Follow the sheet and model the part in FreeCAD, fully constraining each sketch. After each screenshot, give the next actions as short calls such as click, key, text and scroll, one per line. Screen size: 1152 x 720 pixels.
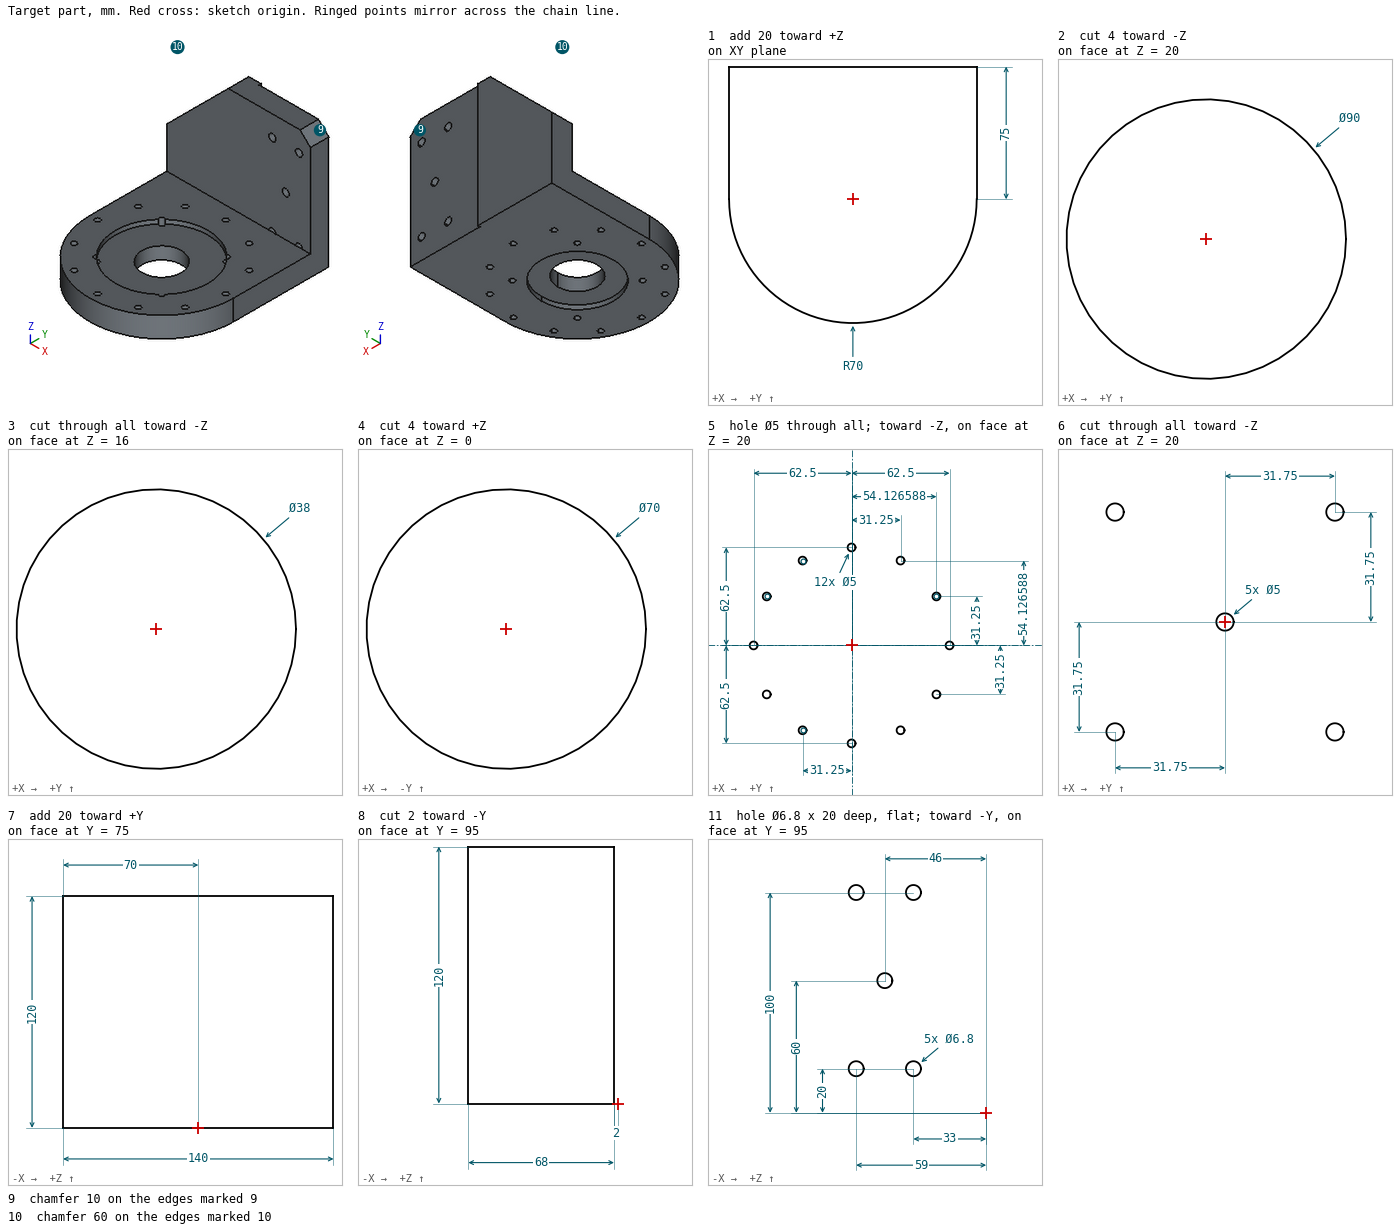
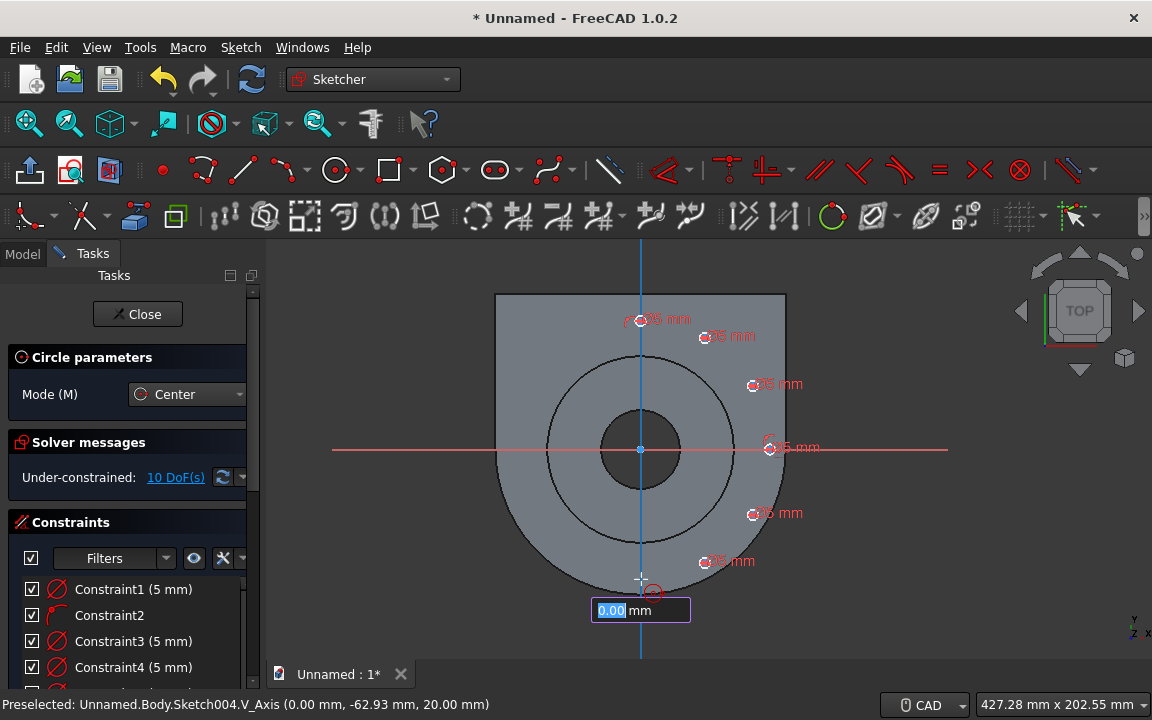
scroll(645, 577, up, 6)
move(645, 576)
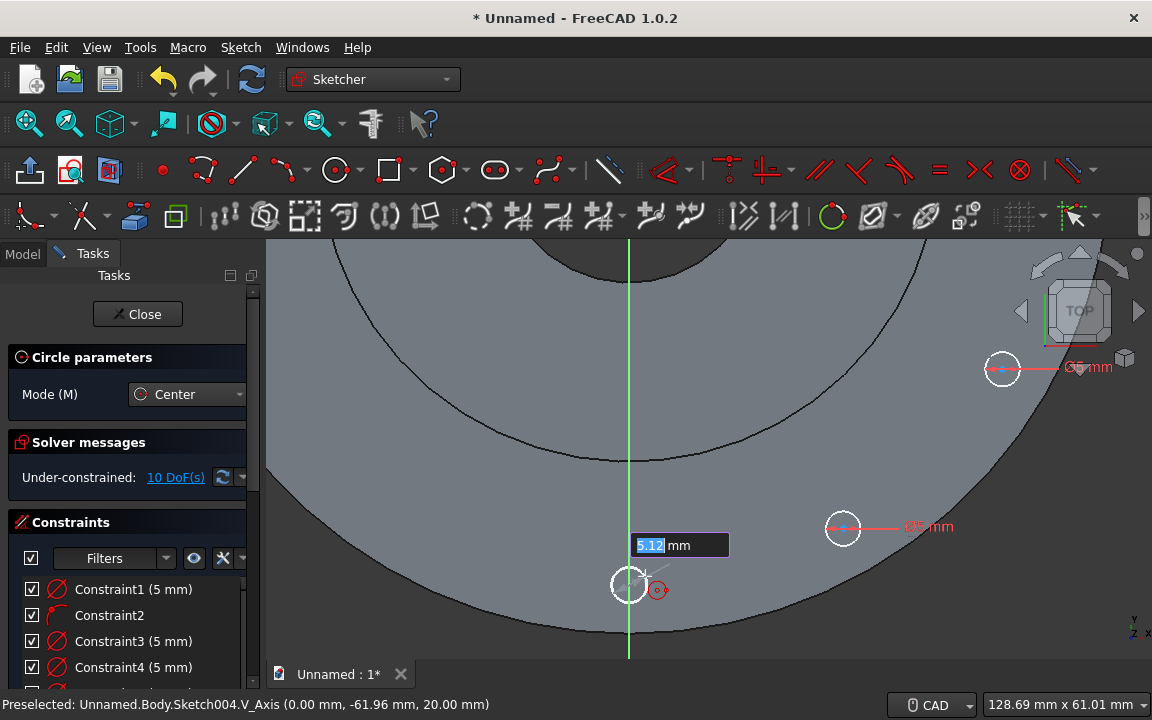
text(5)
key(Return)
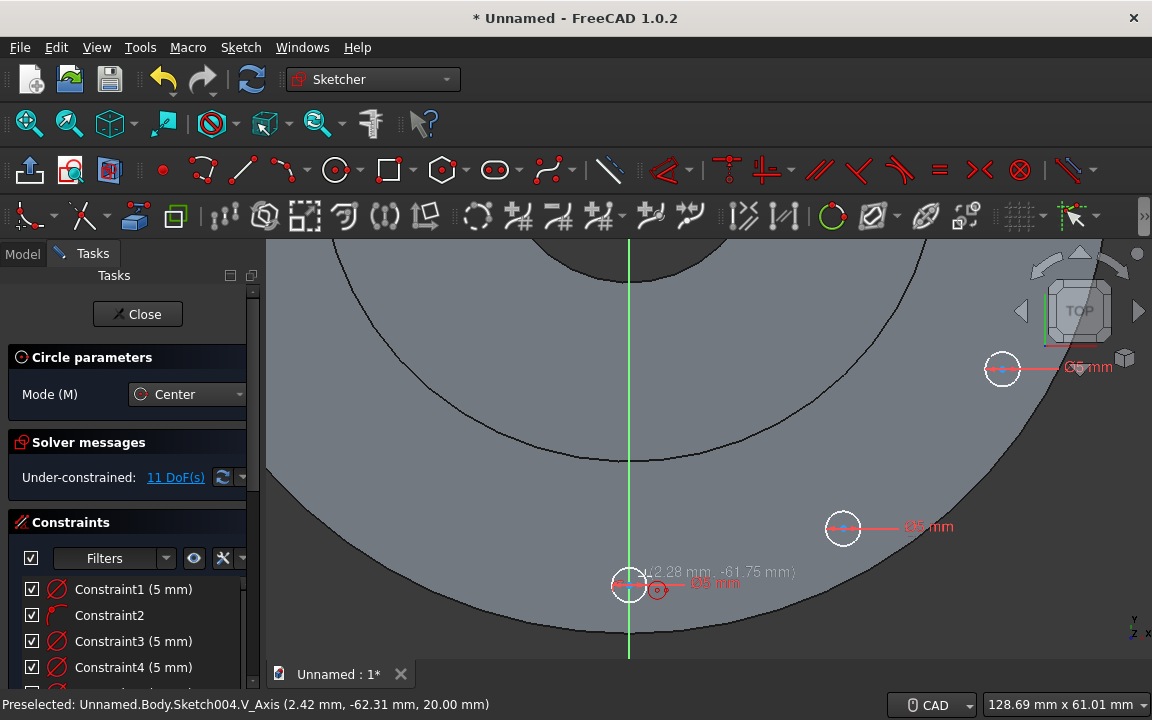
scroll(414, 524, up, 2)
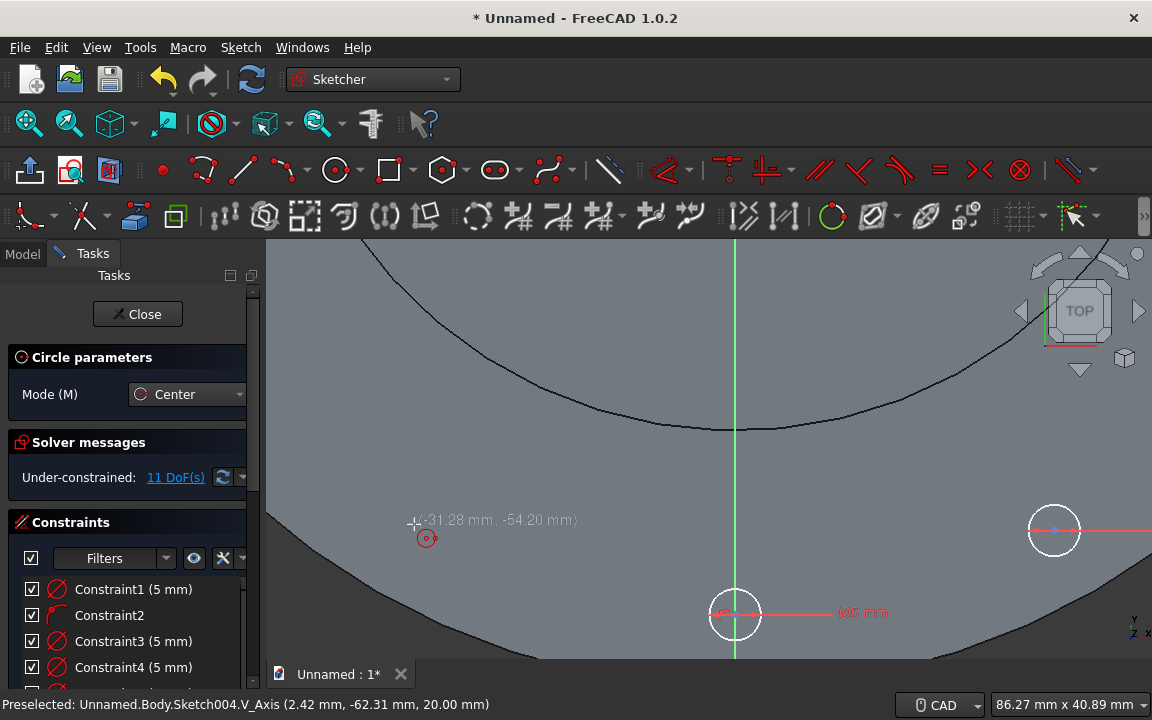
scroll(617, 571, down, 8)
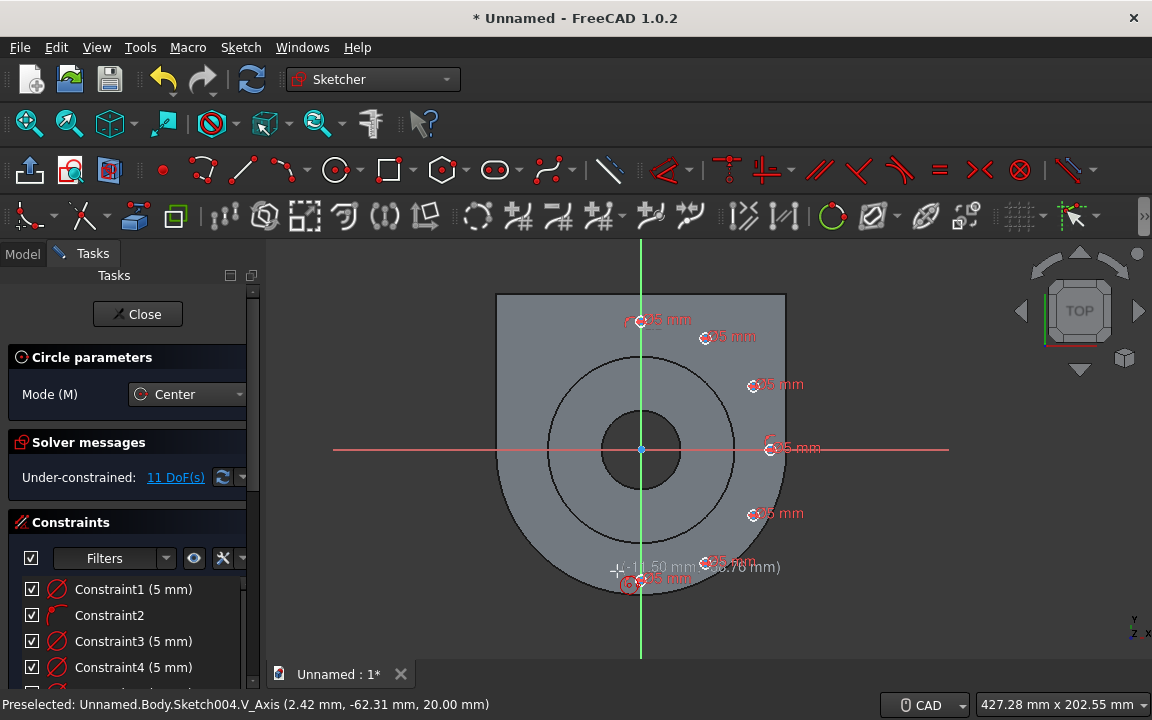
click(576, 562)
move(580, 559)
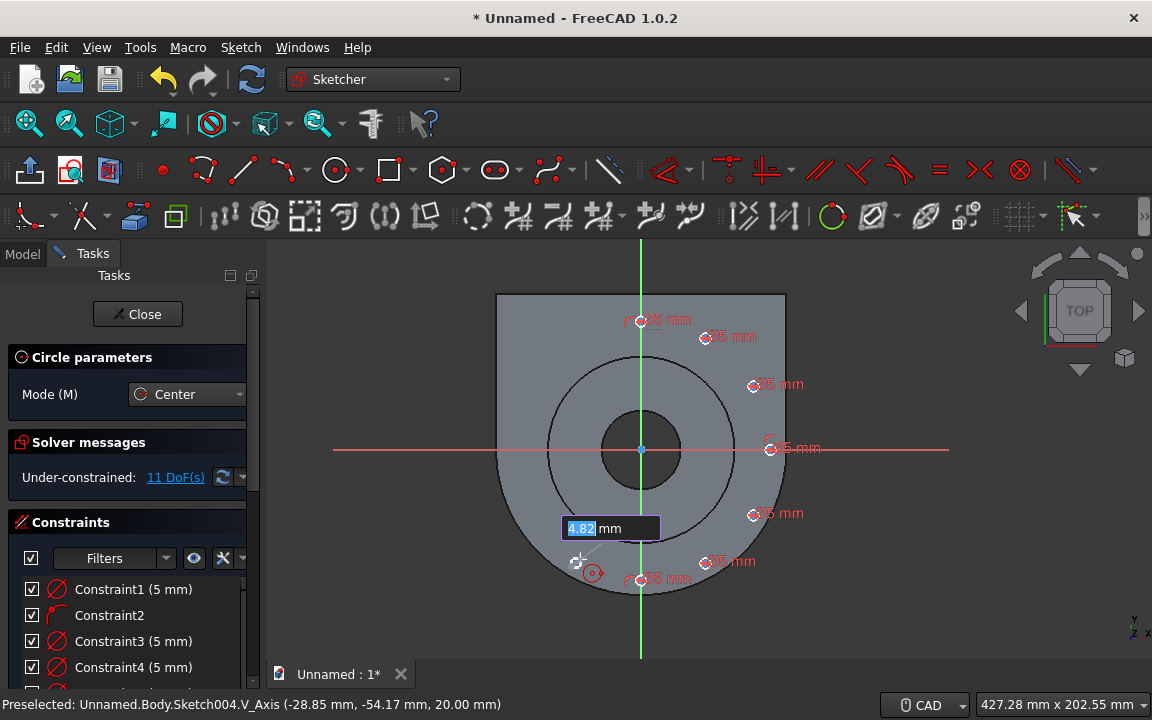
text(5)
key(Return)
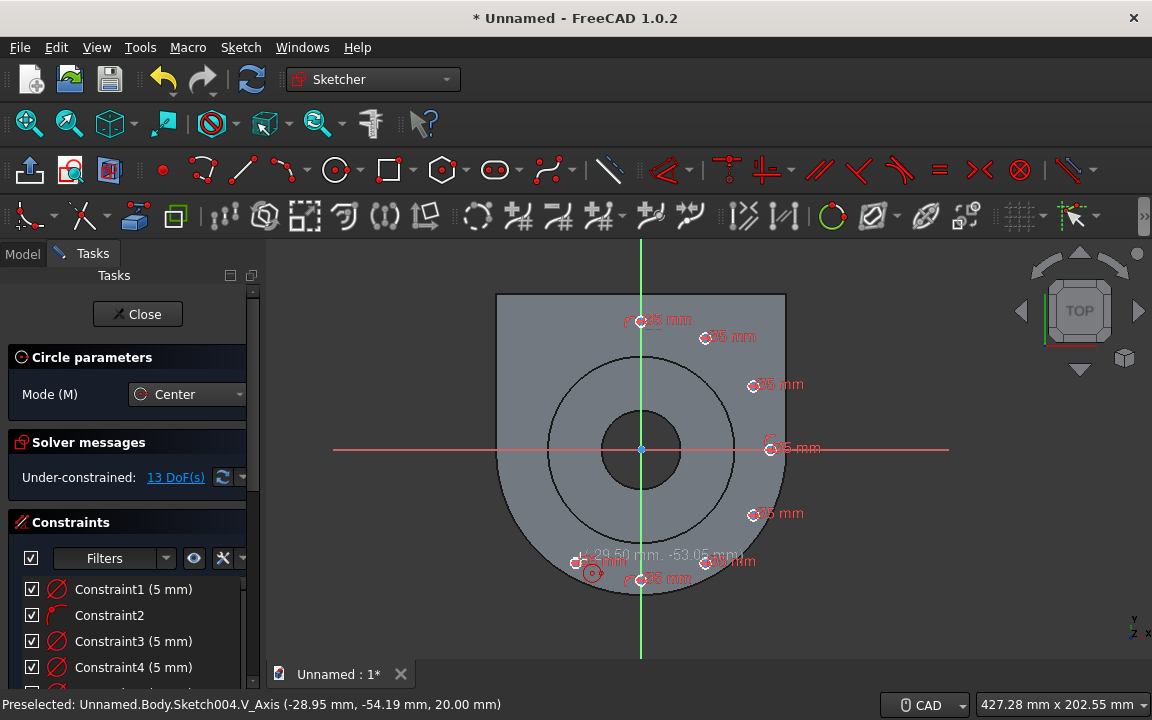
scroll(529, 515, up, 8)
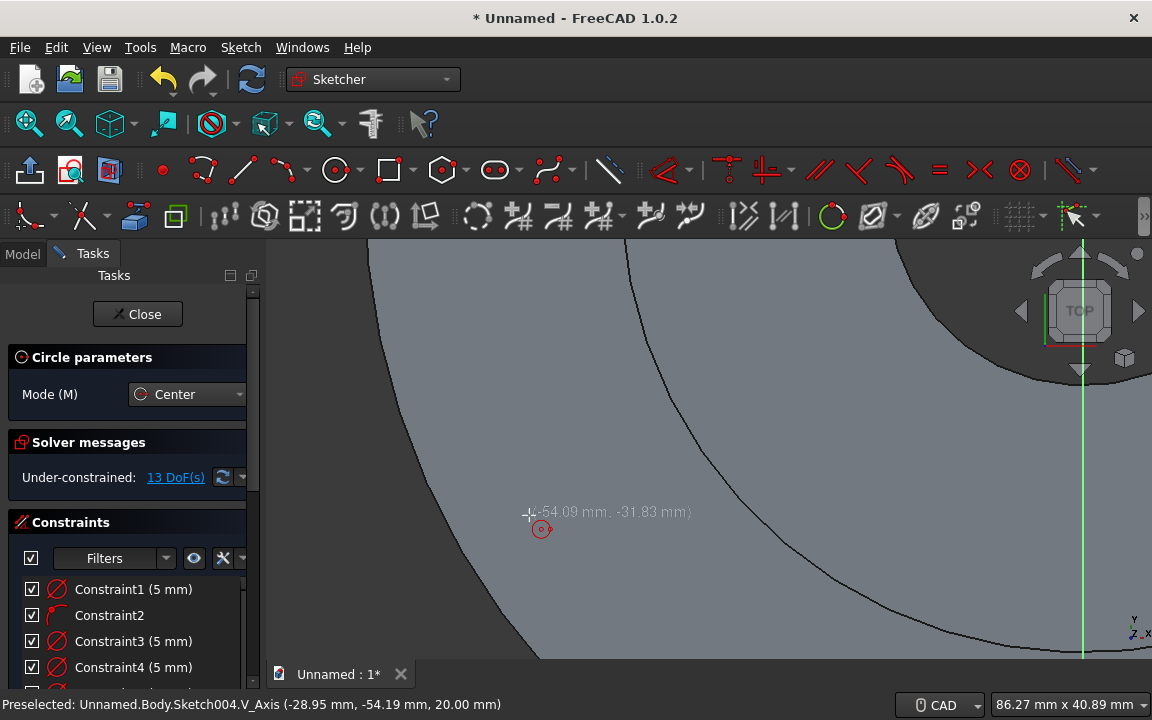
scroll(528, 514, down, 8)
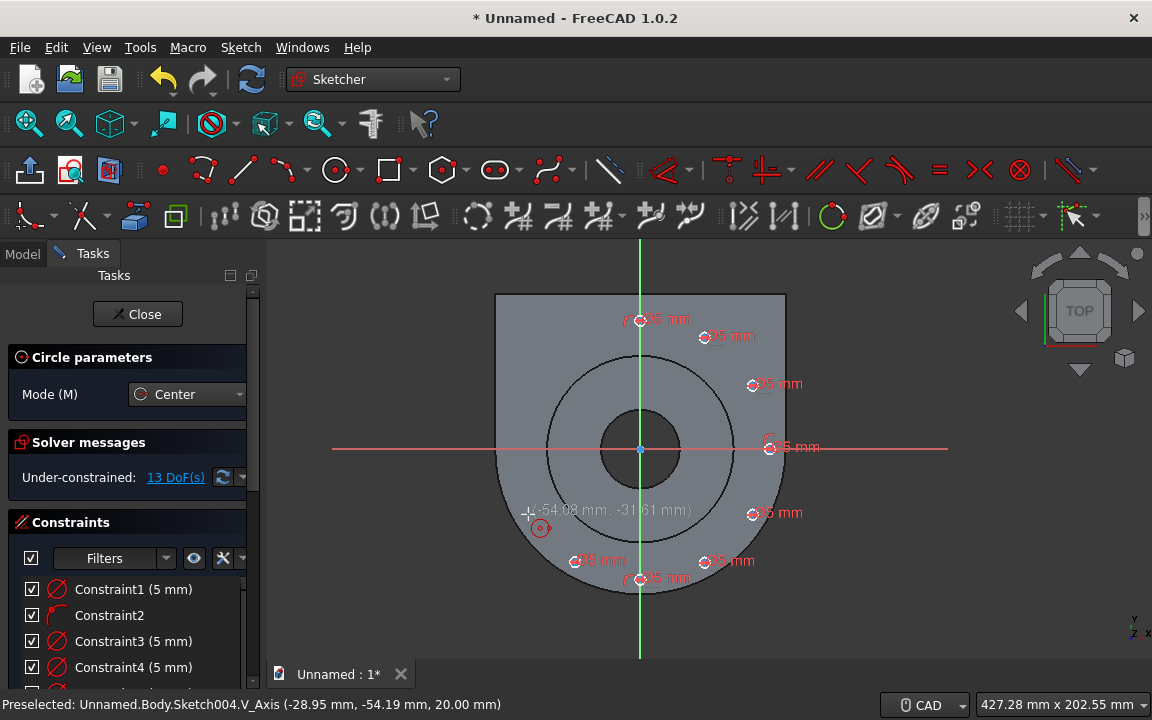
click(528, 514)
move(532, 510)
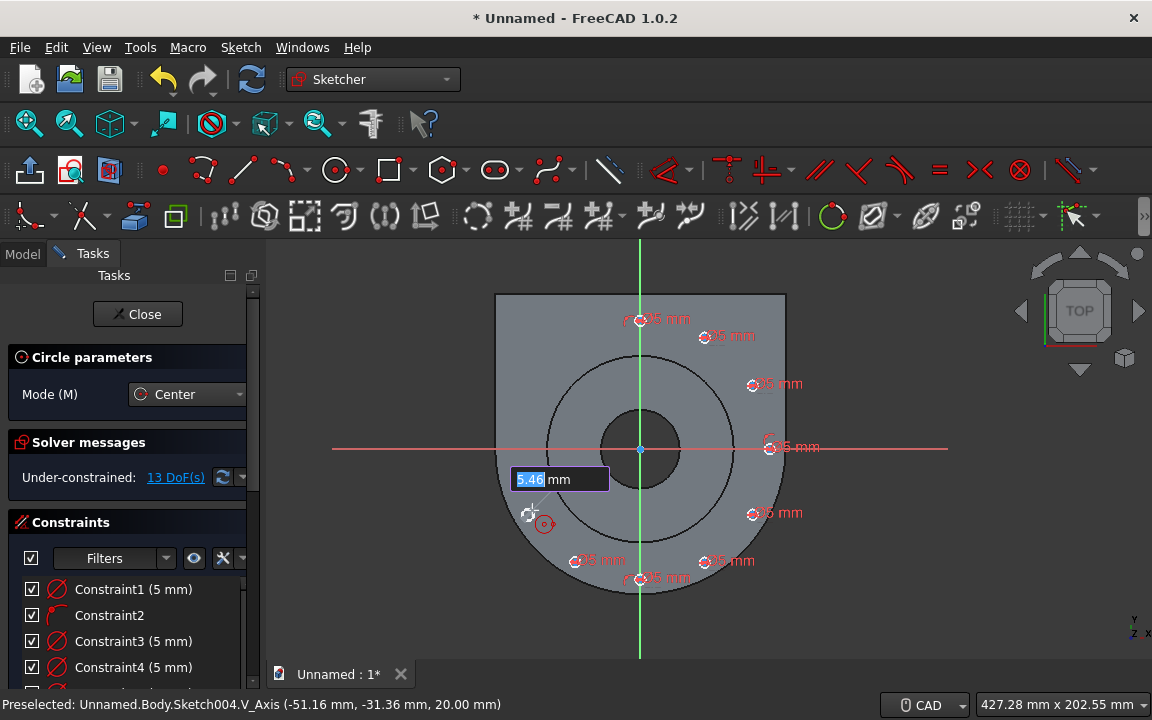
text(5)
key(Return)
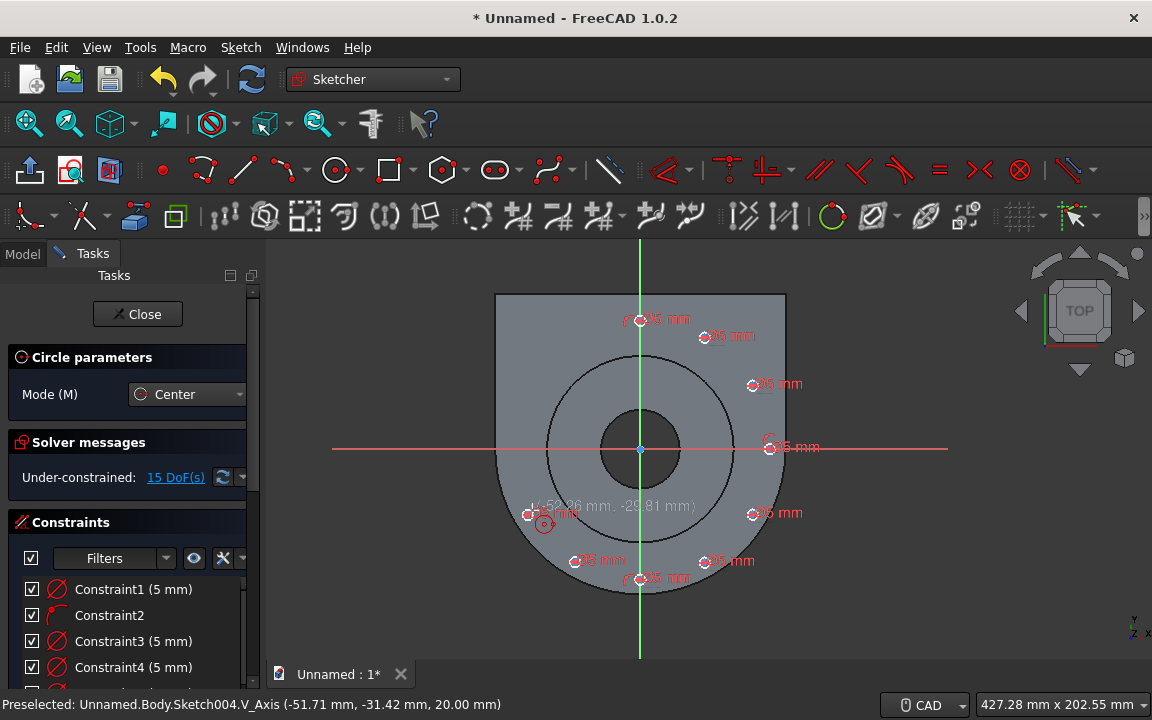
scroll(511, 449, up, 8)